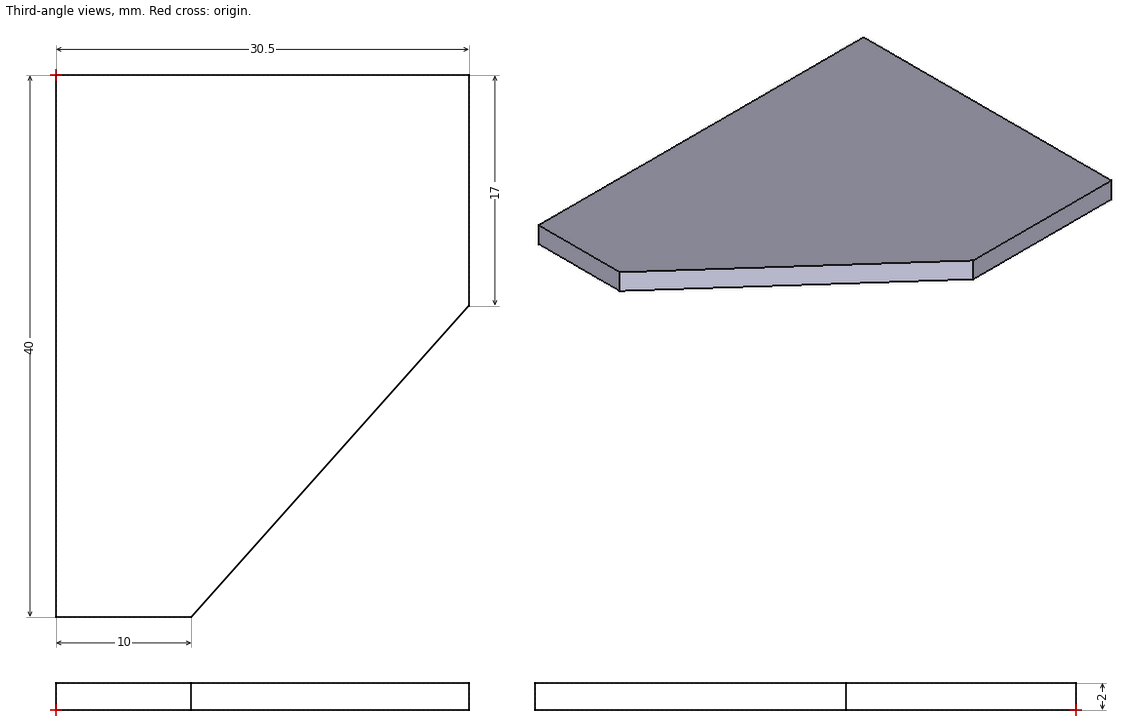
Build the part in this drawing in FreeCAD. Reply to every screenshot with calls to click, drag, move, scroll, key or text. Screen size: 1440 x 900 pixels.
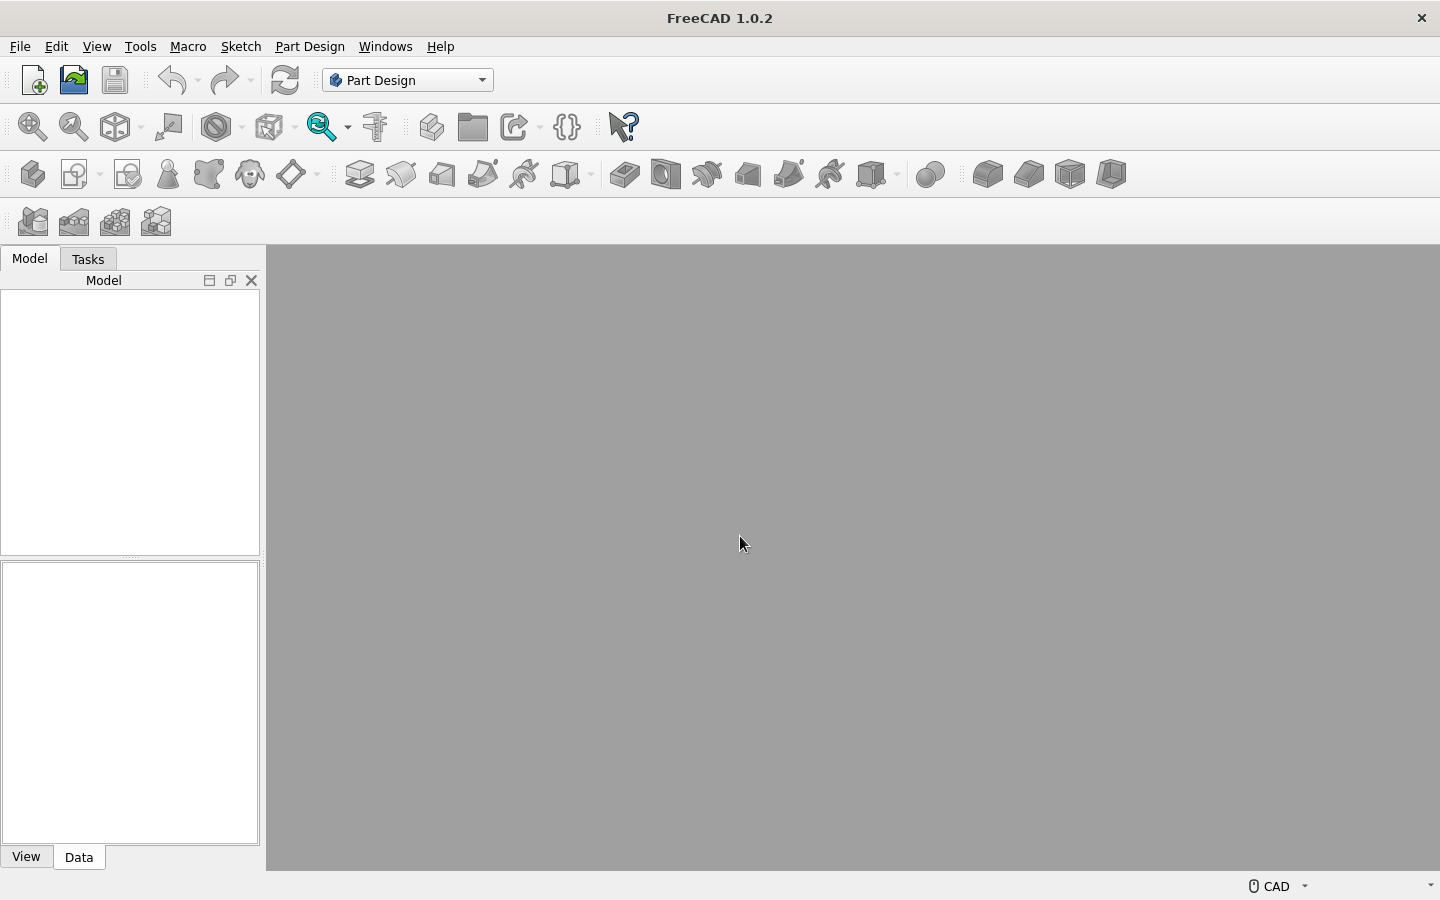
key(ctrl+n)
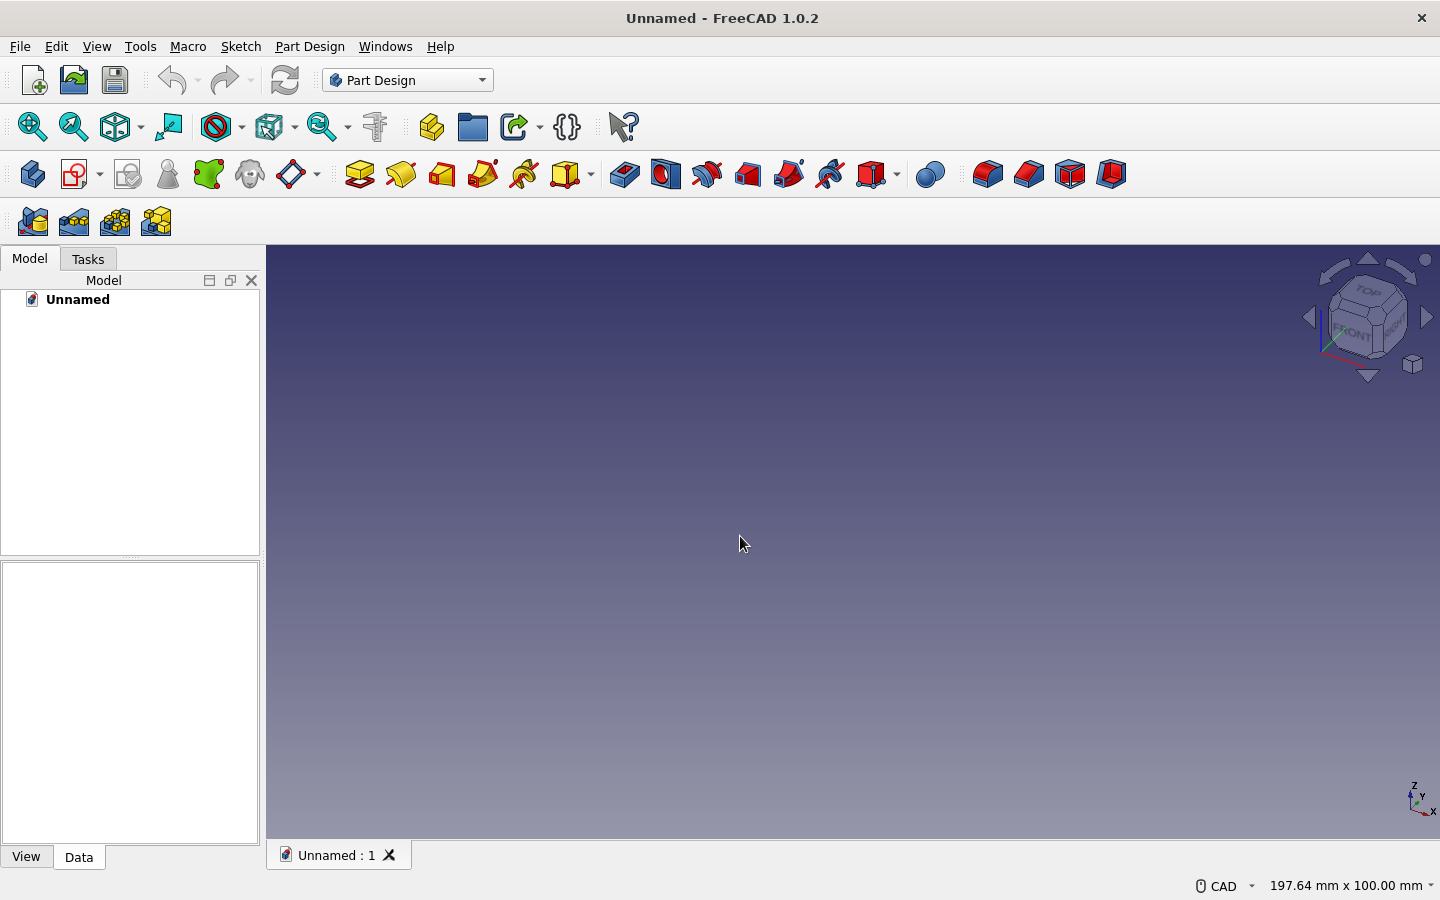
click(74, 174)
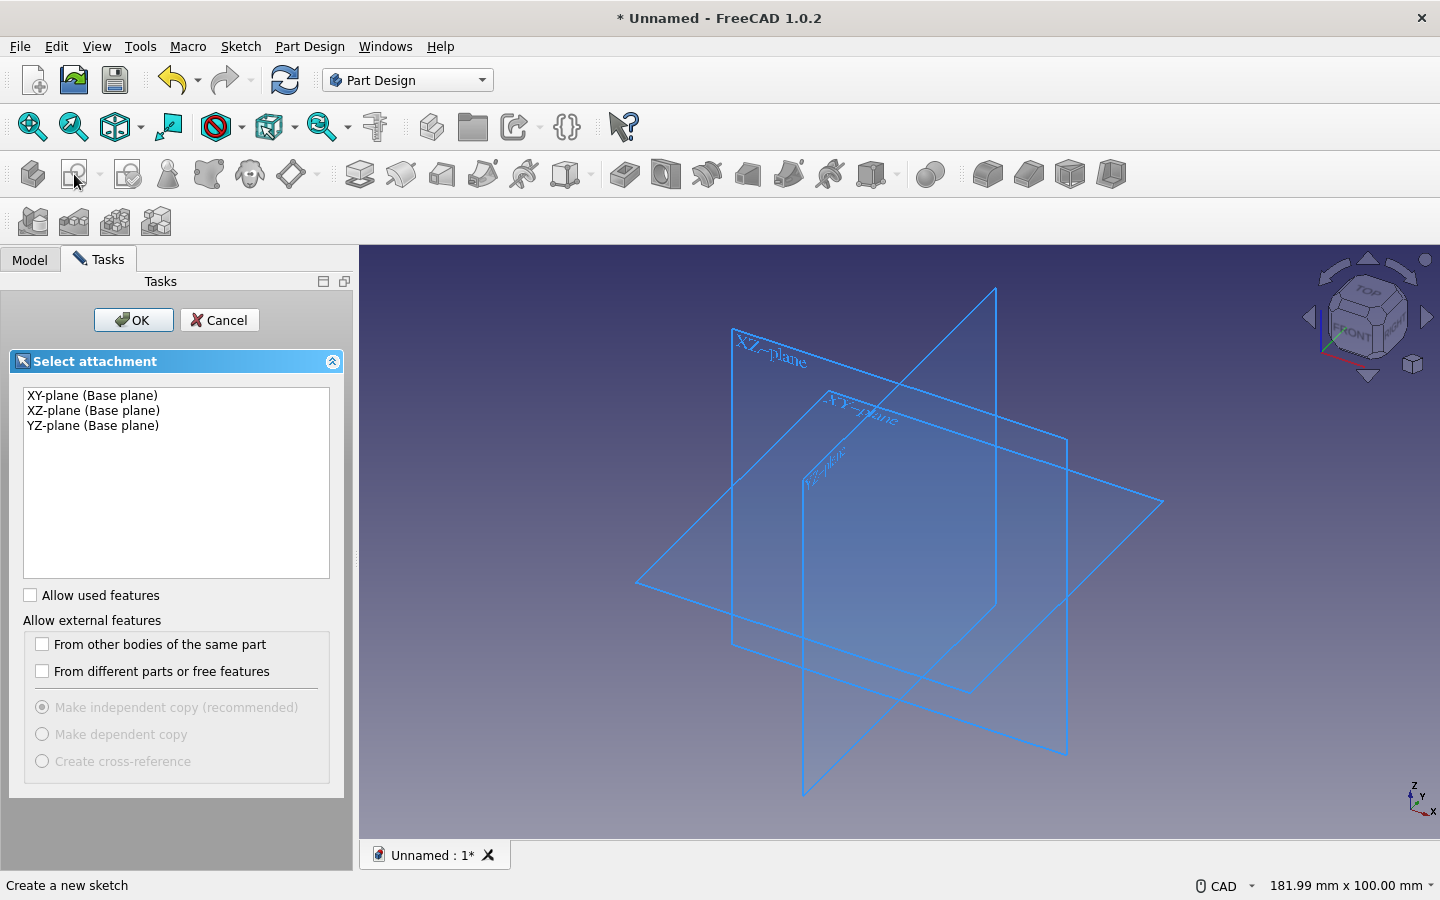
click(84, 396)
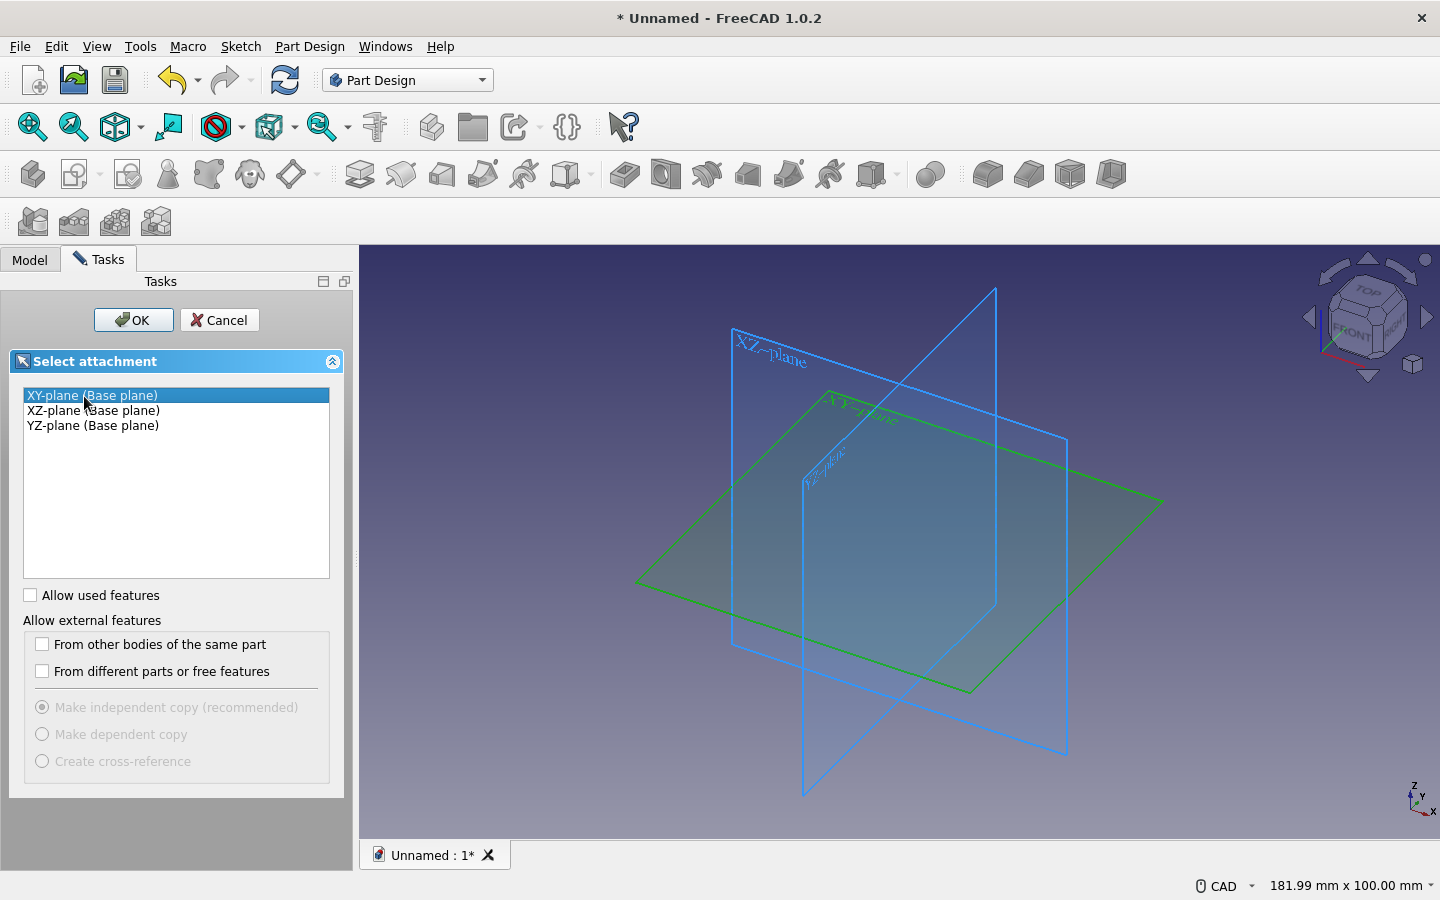
click(134, 320)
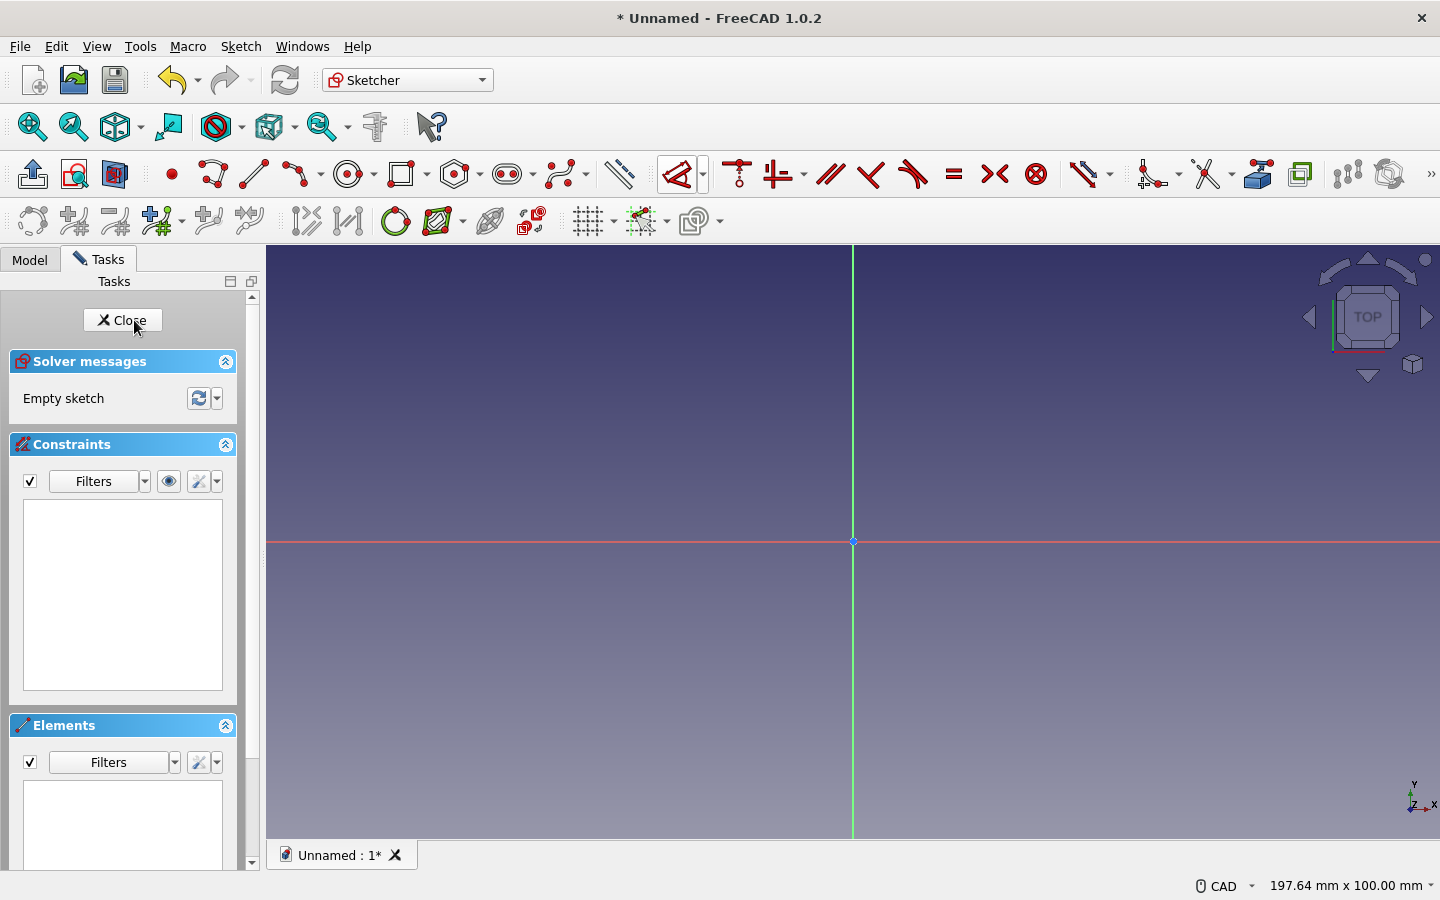
scroll(1267, 811, up, 2)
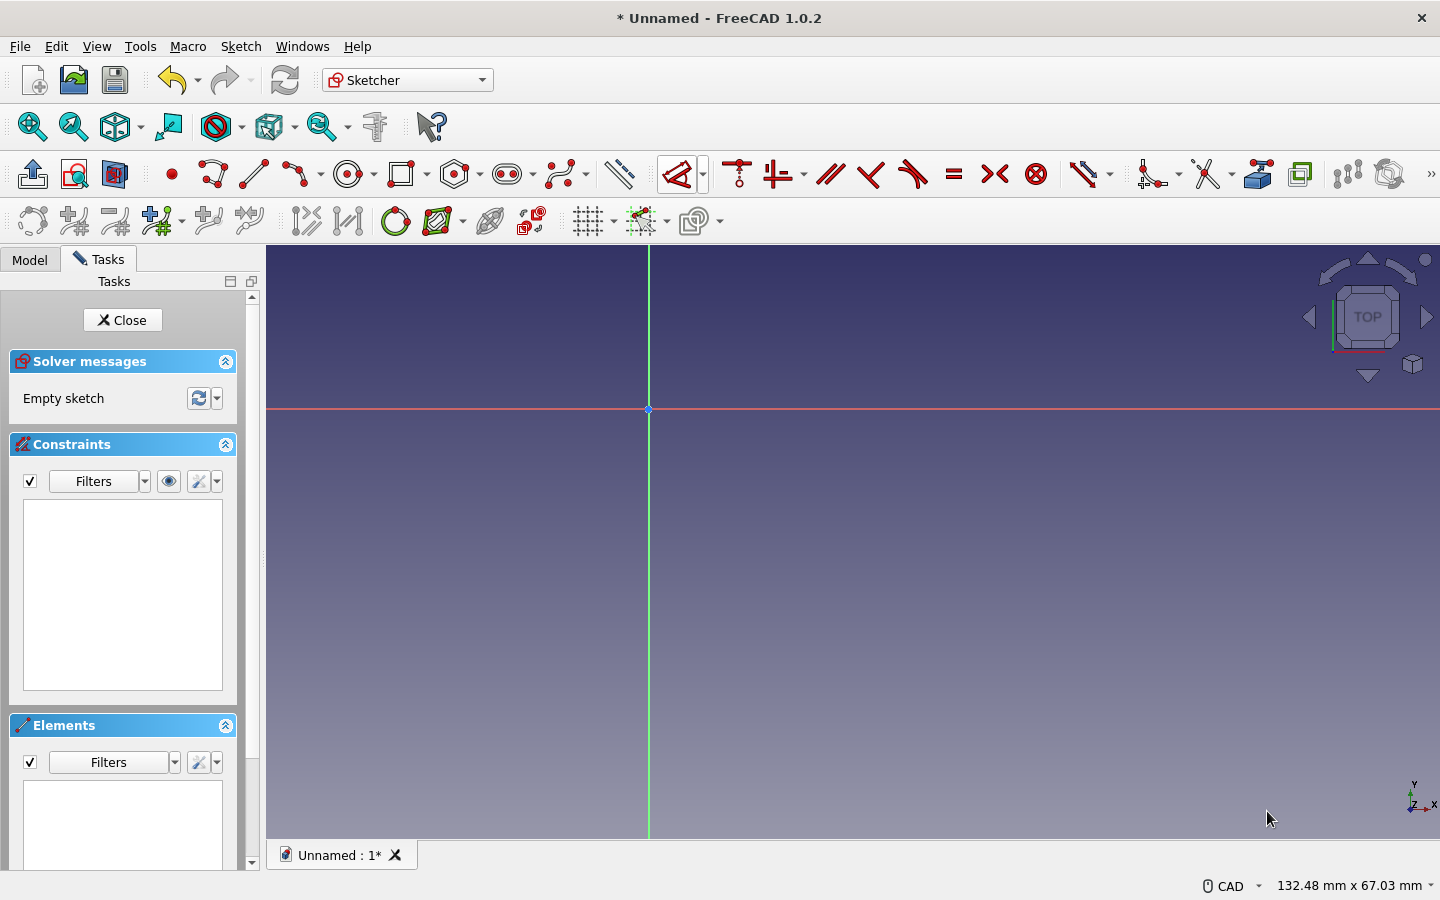
key(g)
key(m)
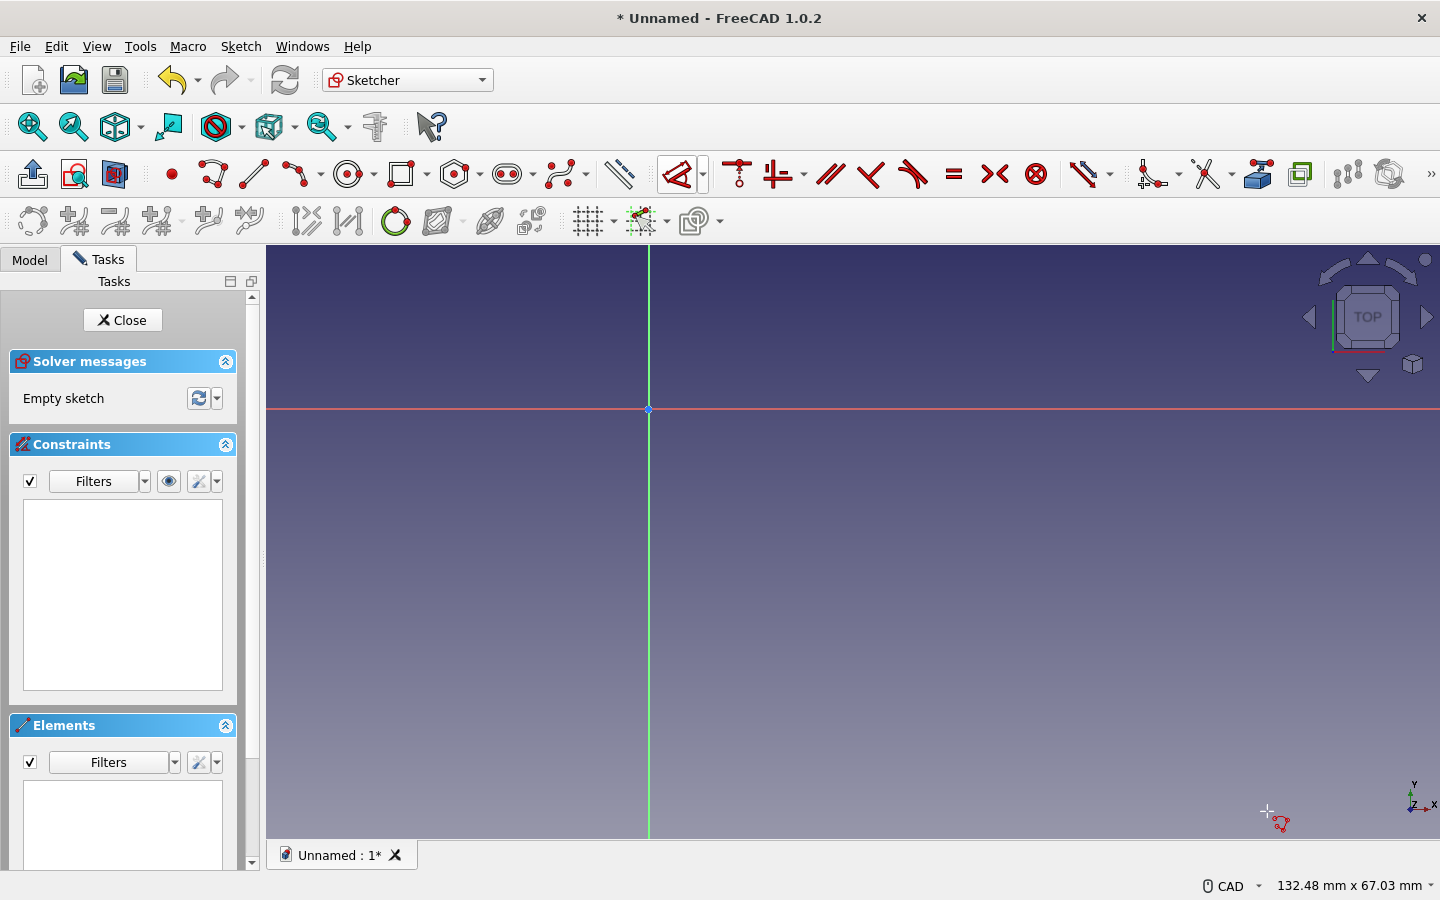
click(649, 409)
click(658, 764)
click(738, 764)
click(919, 560)
click(919, 418)
click(649, 409)
key(Escape)
key(Escape)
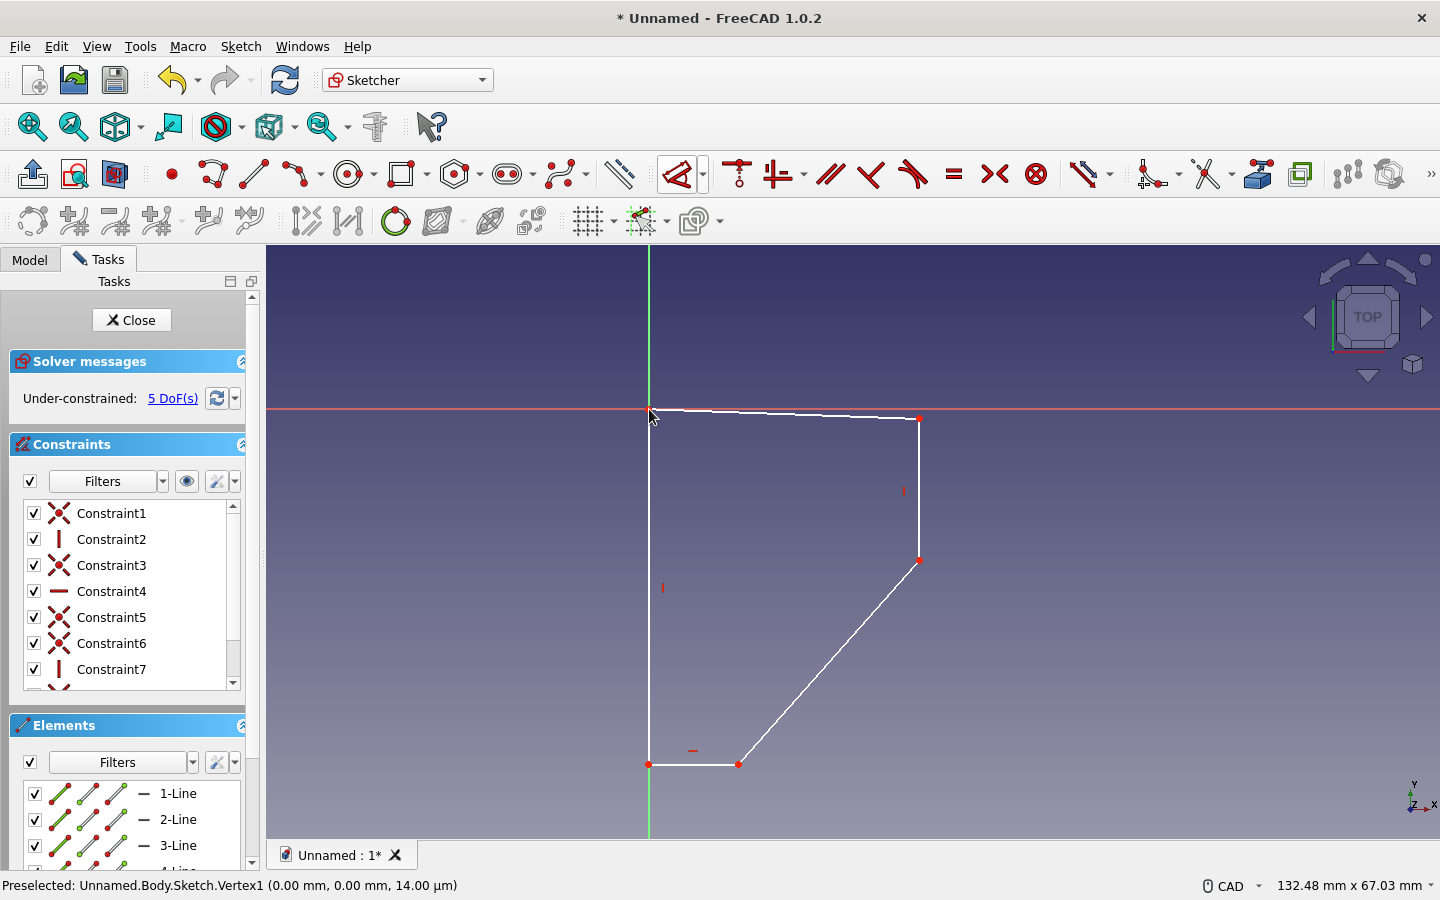
click(730, 412)